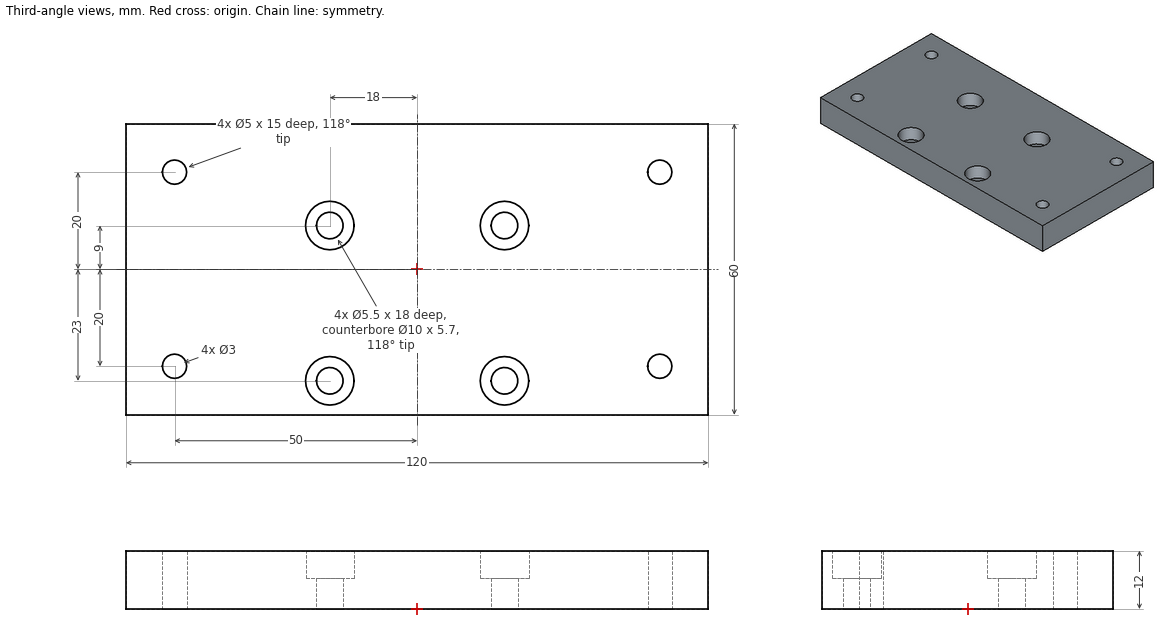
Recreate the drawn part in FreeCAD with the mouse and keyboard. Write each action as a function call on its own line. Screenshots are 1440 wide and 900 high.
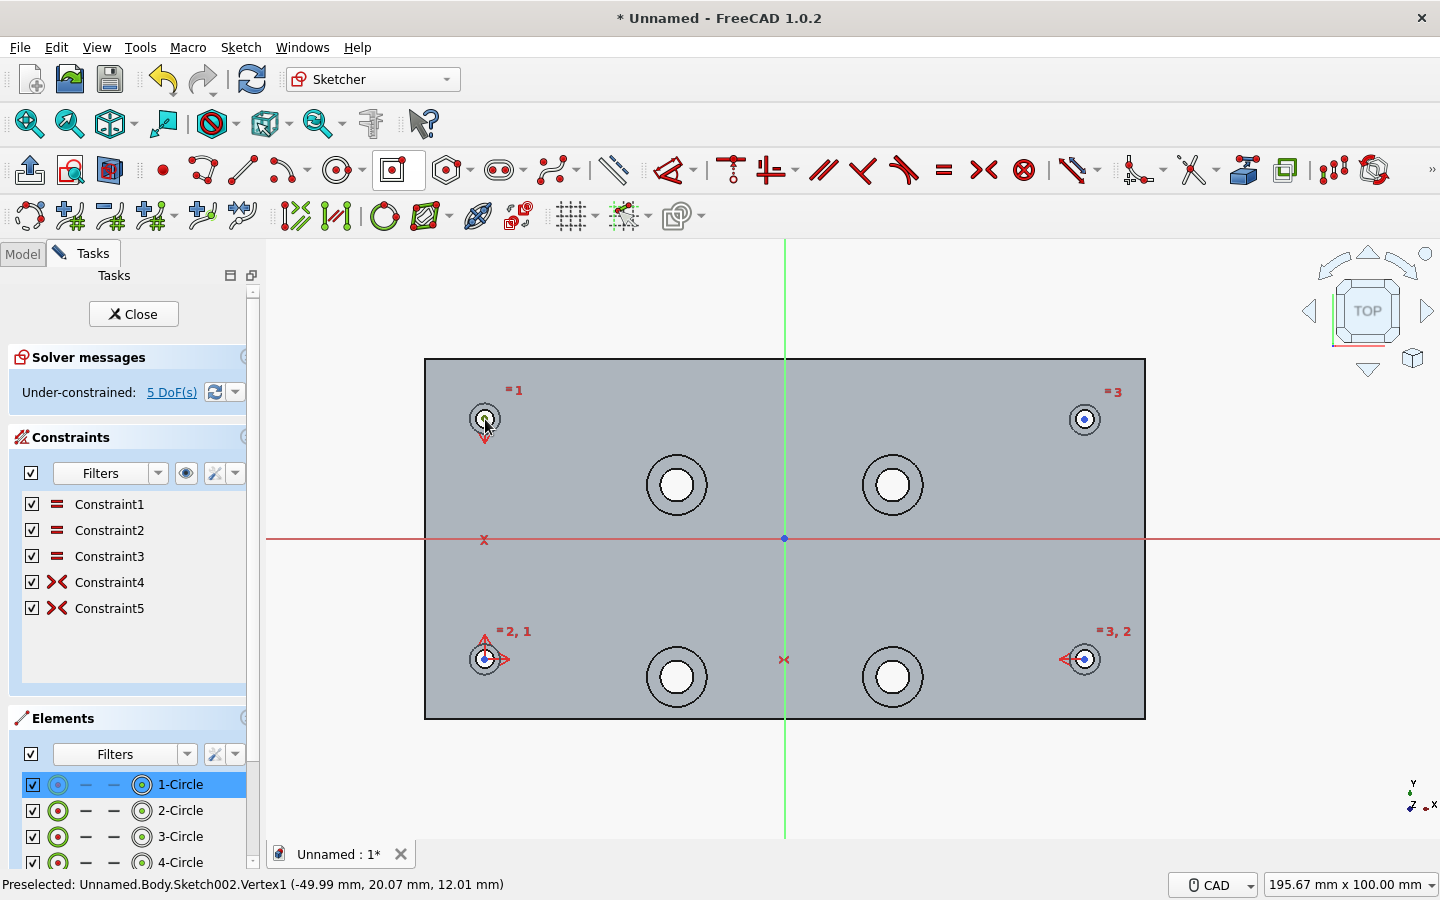
click(1085, 420)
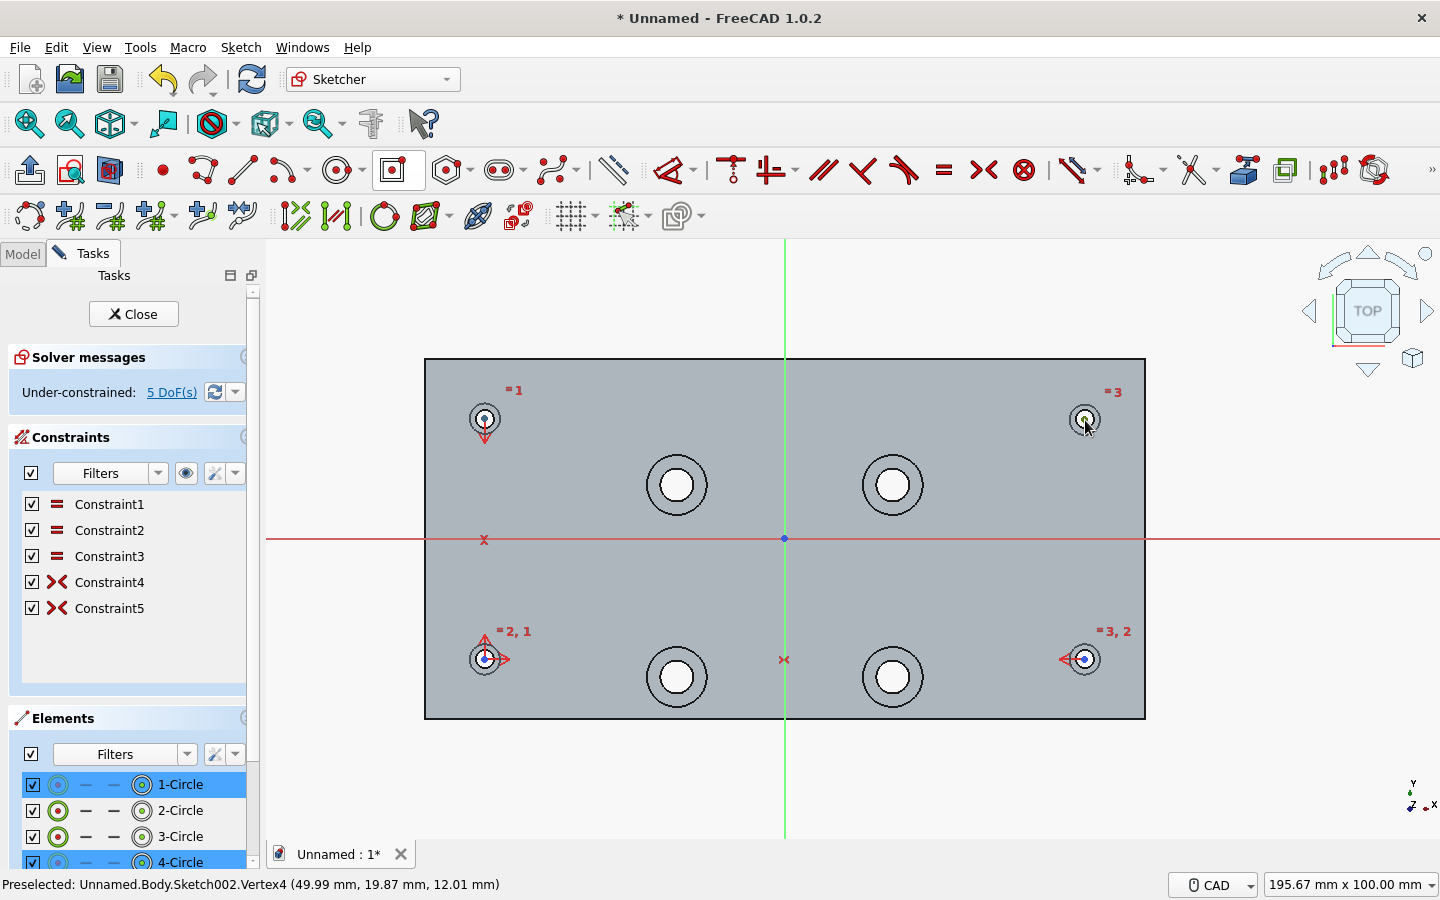
click(785, 772)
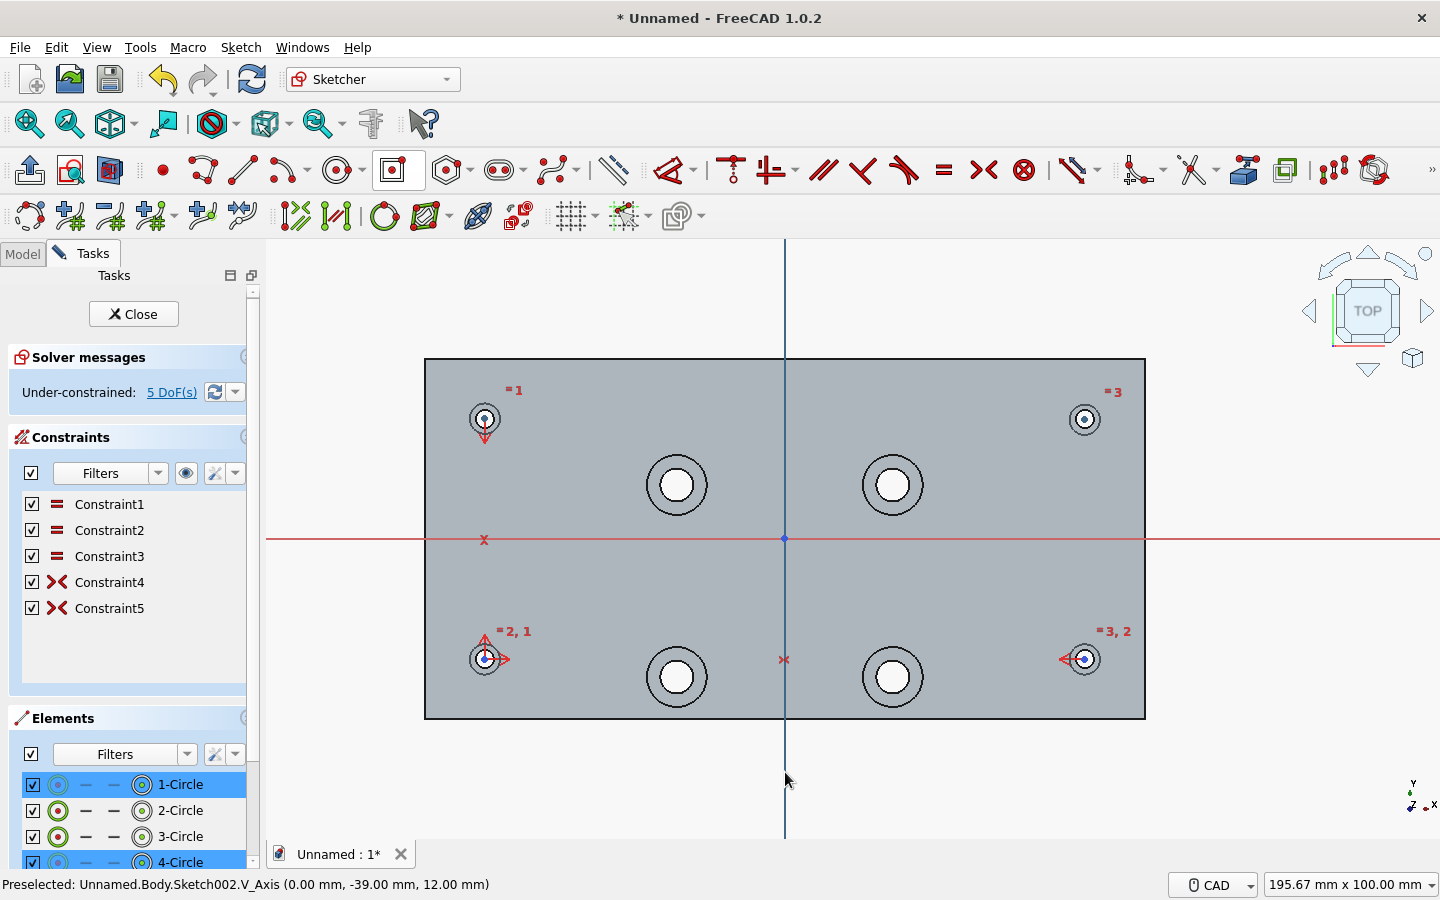
click(984, 170)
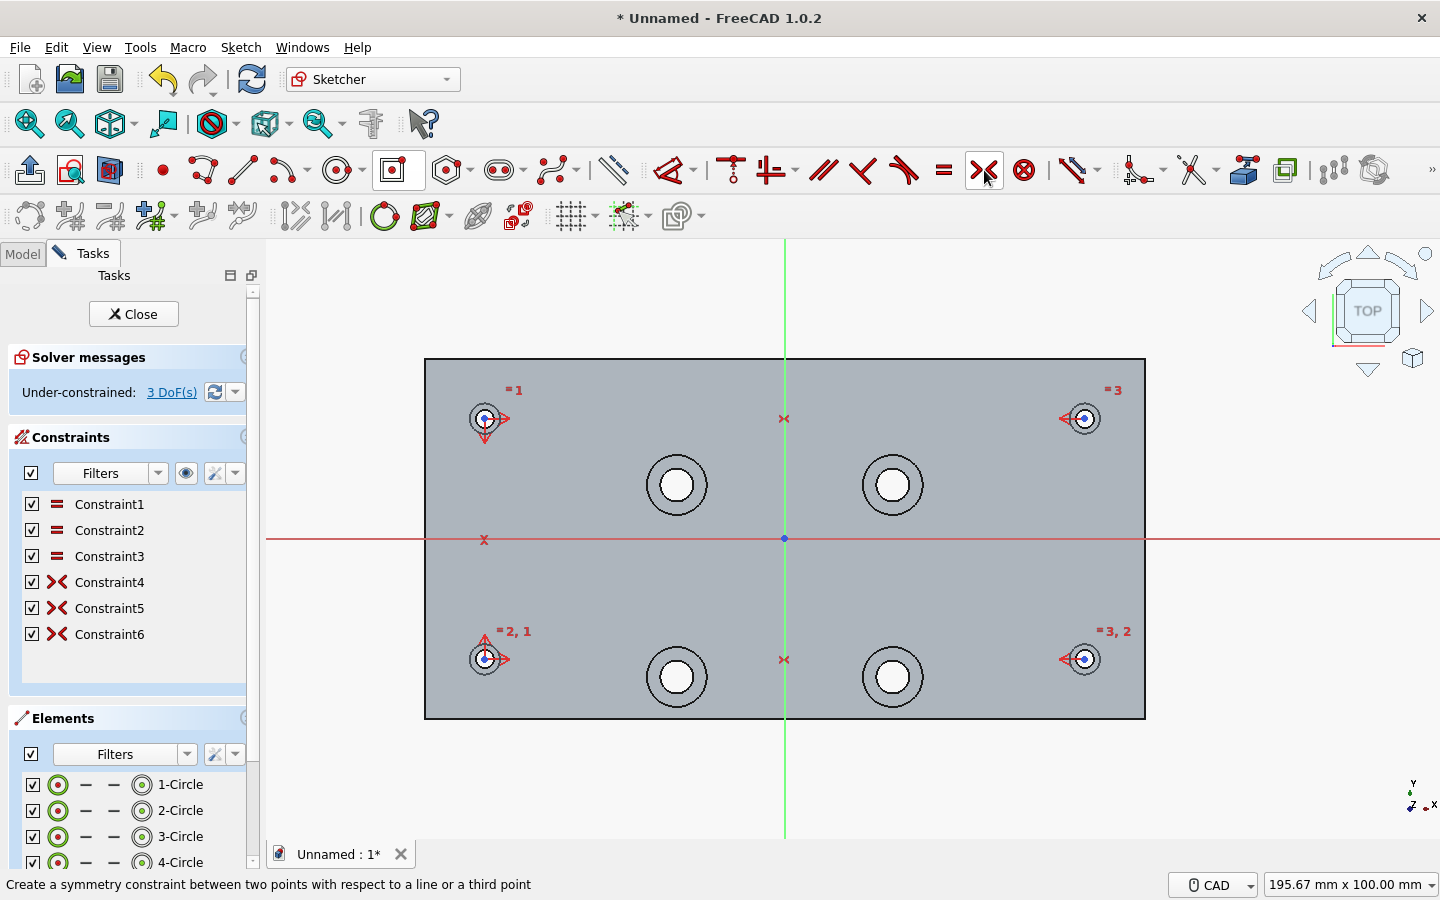
click(668, 170)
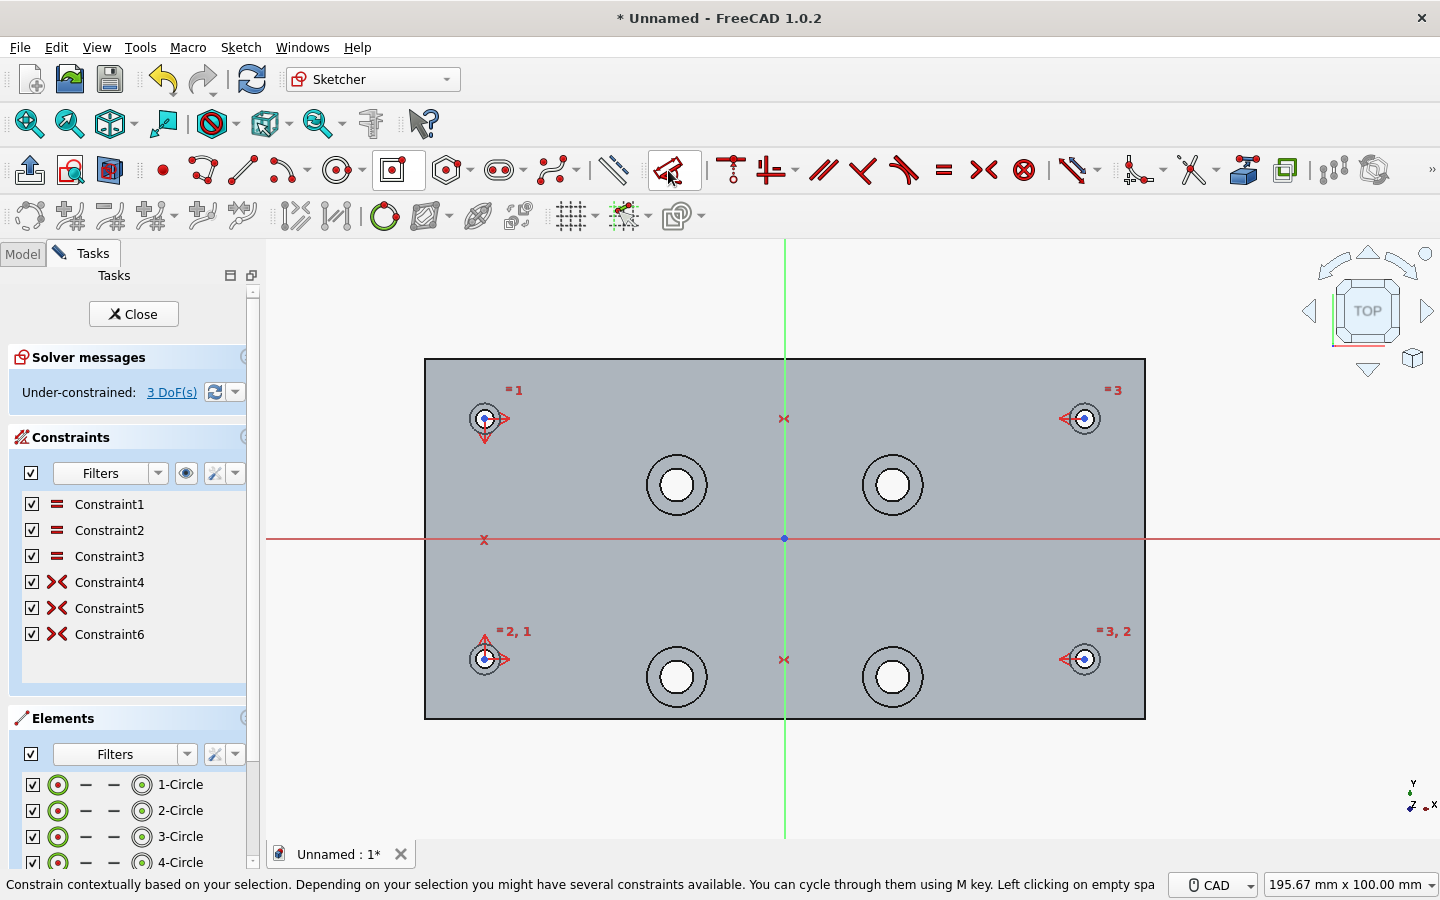
scroll(496, 408, up, 2)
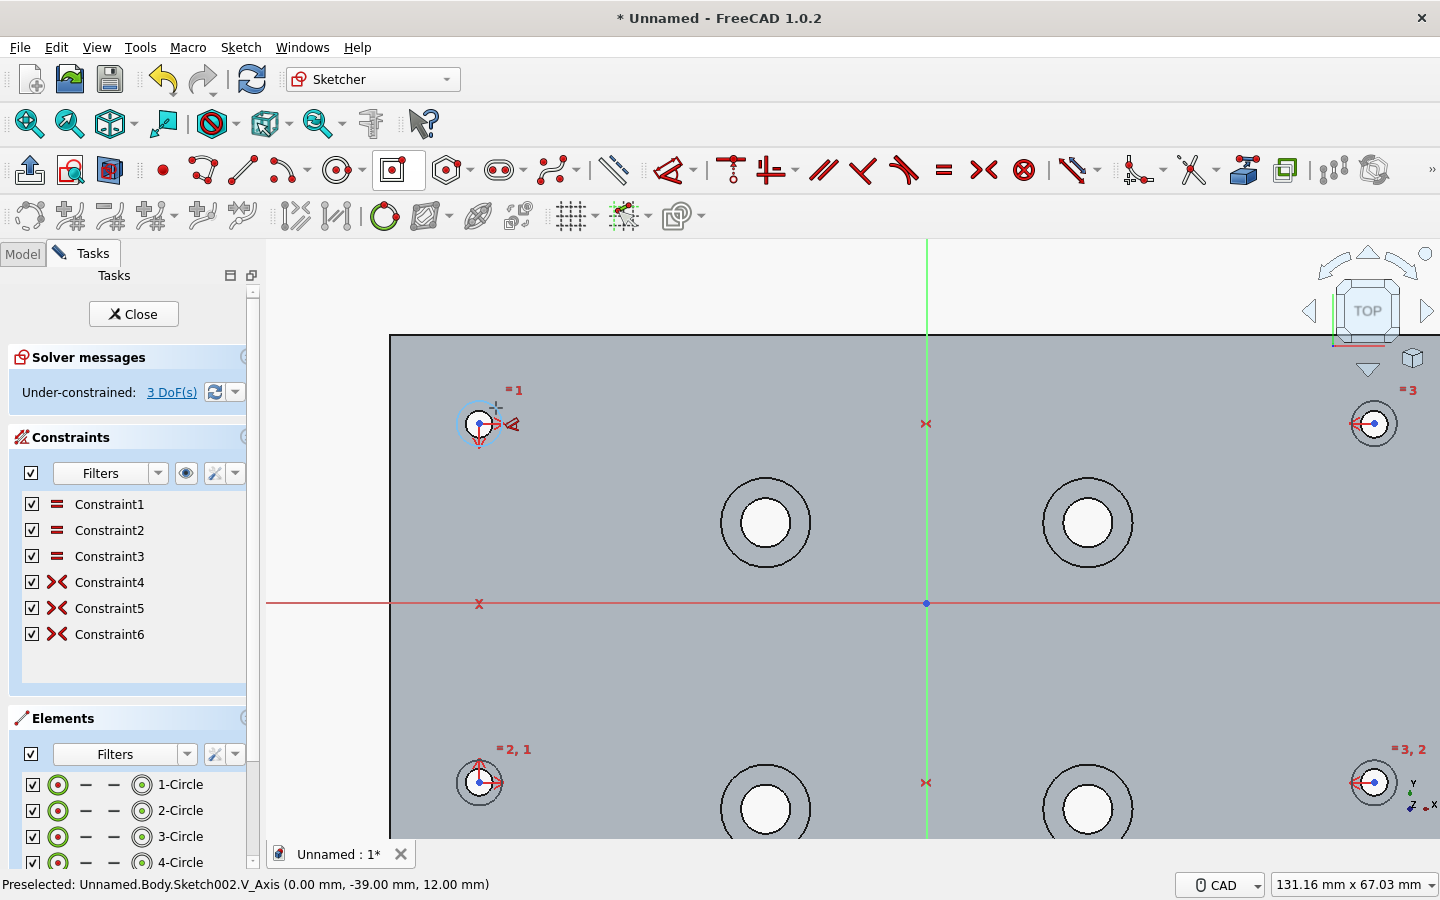
click(495, 408)
click(518, 385)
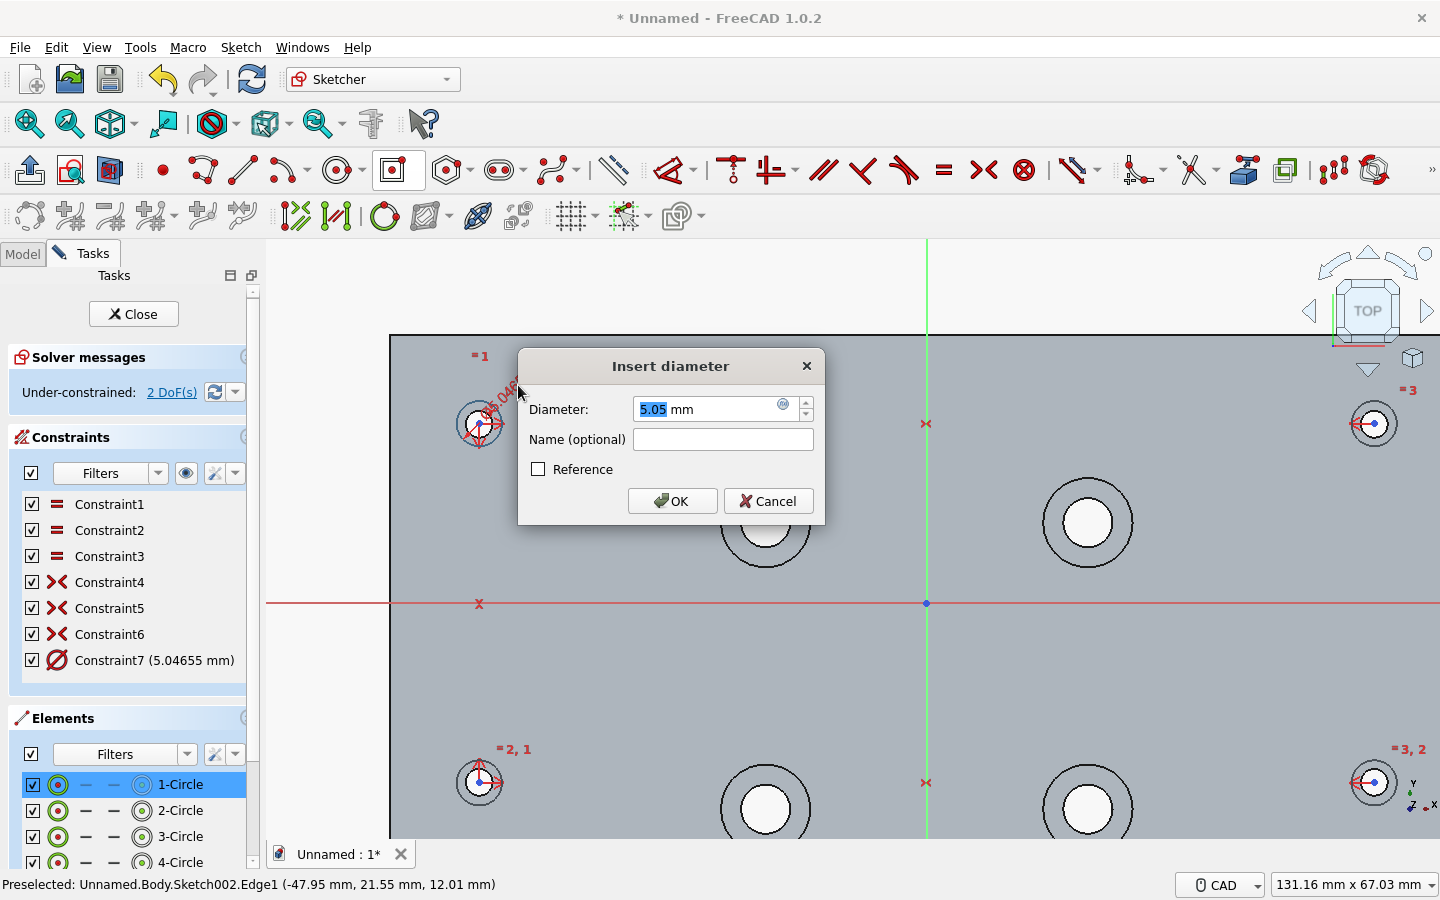
text(5)
key(Return)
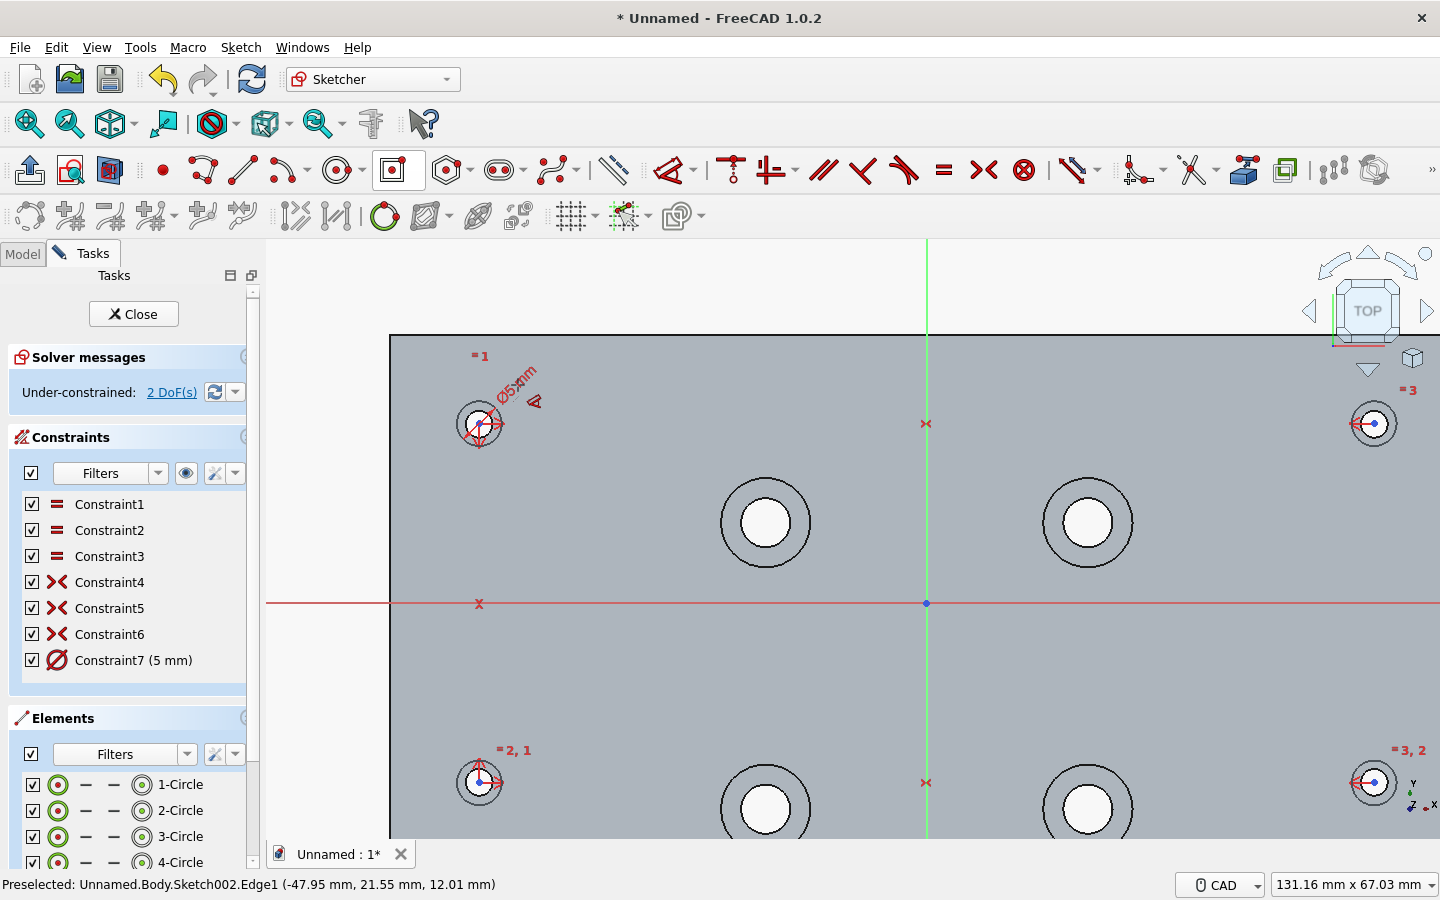
click(479, 424)
click(703, 390)